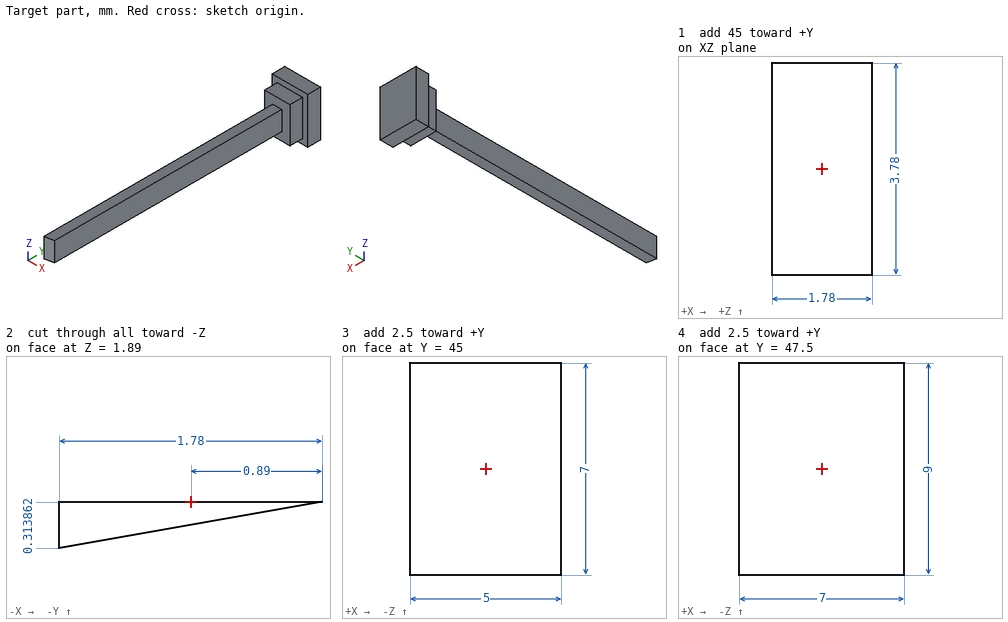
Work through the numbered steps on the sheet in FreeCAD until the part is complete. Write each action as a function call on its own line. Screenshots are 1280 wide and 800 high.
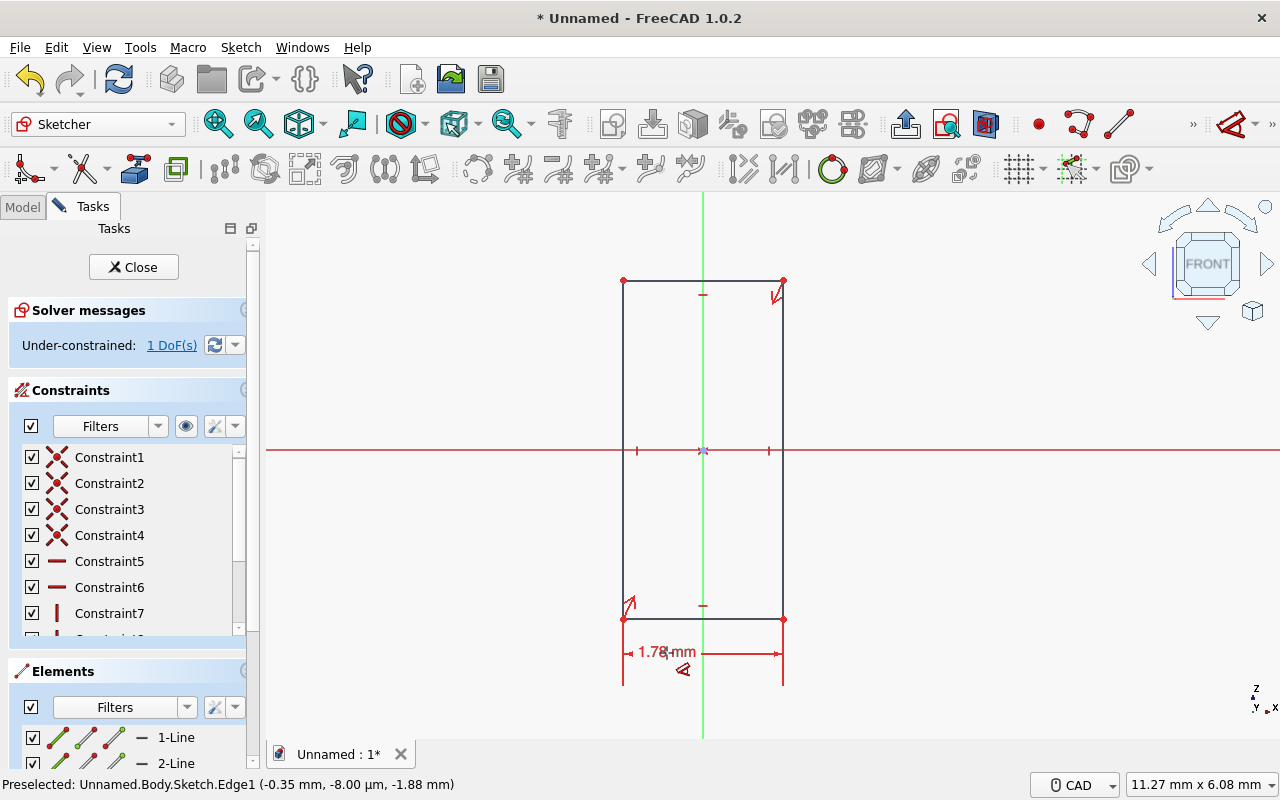
click(783, 518)
click(817, 372)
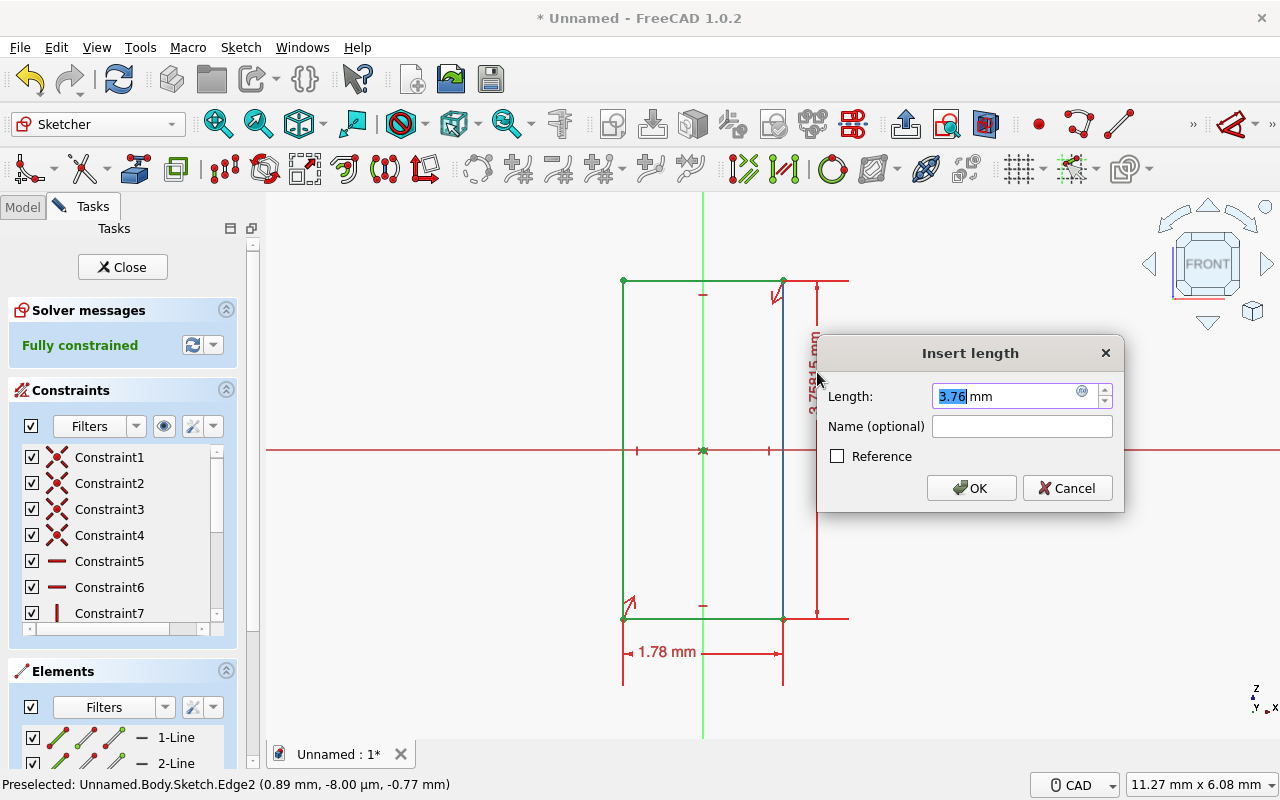
text(3.78)
key(Return)
key(Escape)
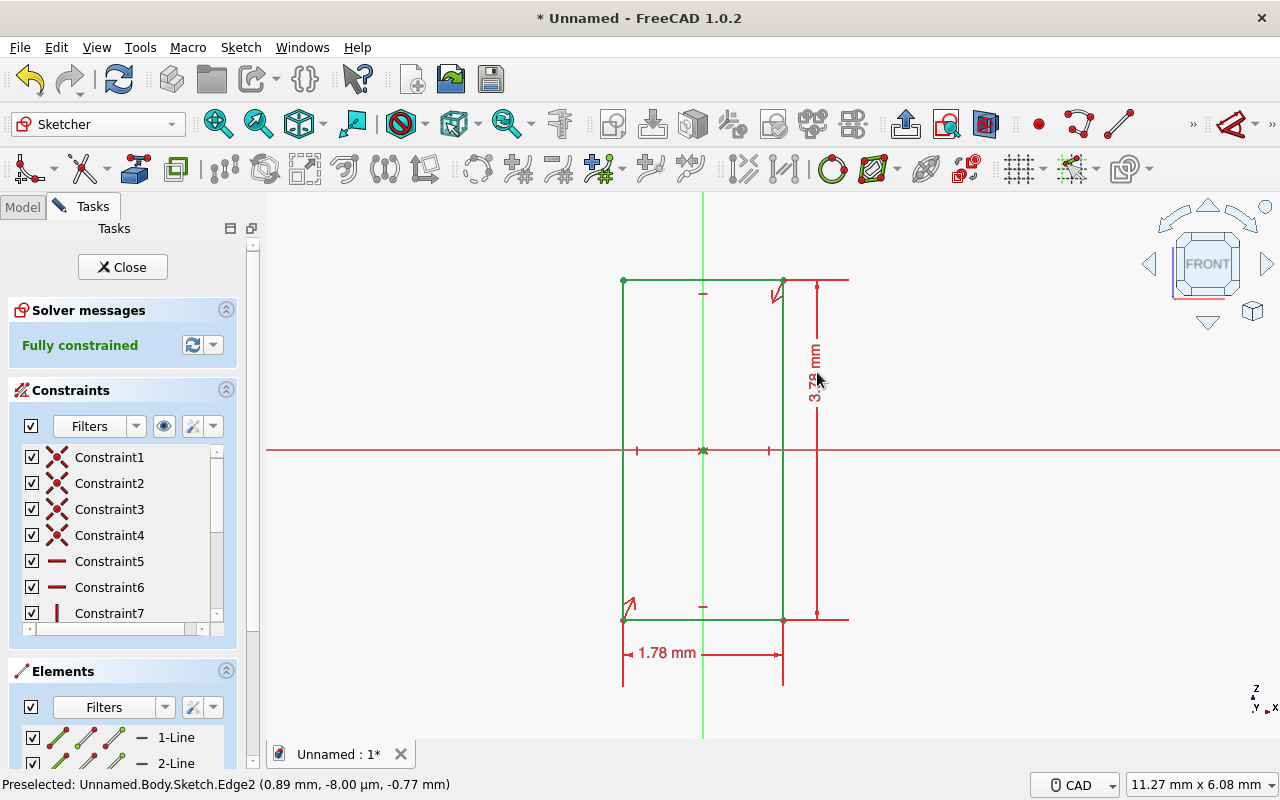
click(123, 267)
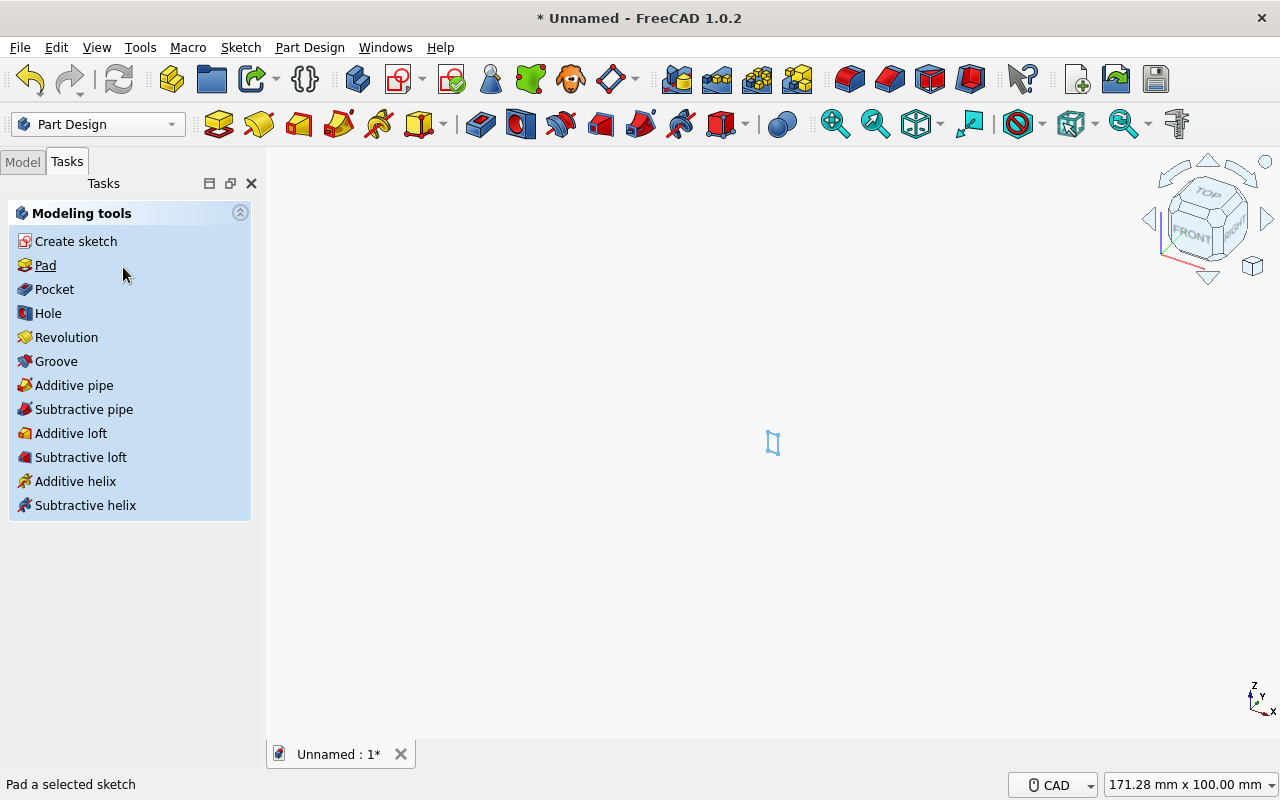
click(220, 124)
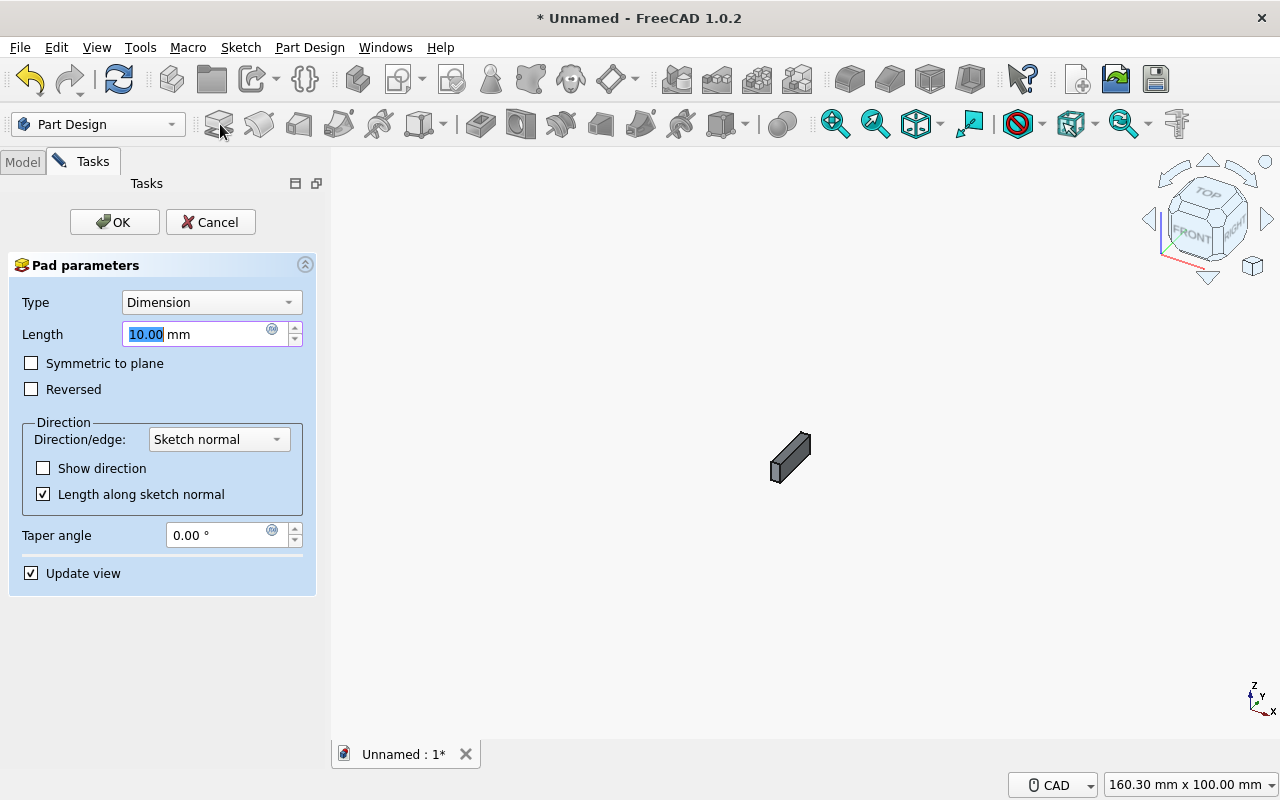
text(45)
key(Tab)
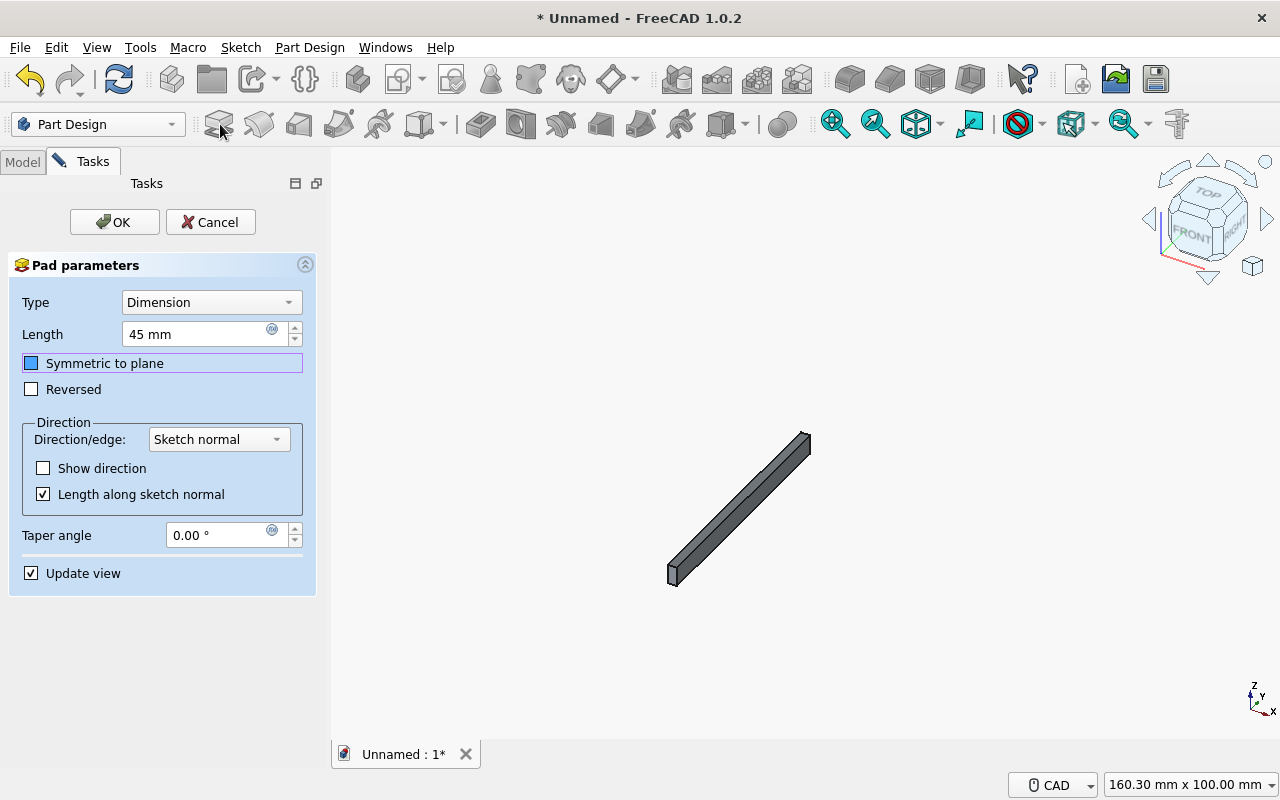
click(30, 389)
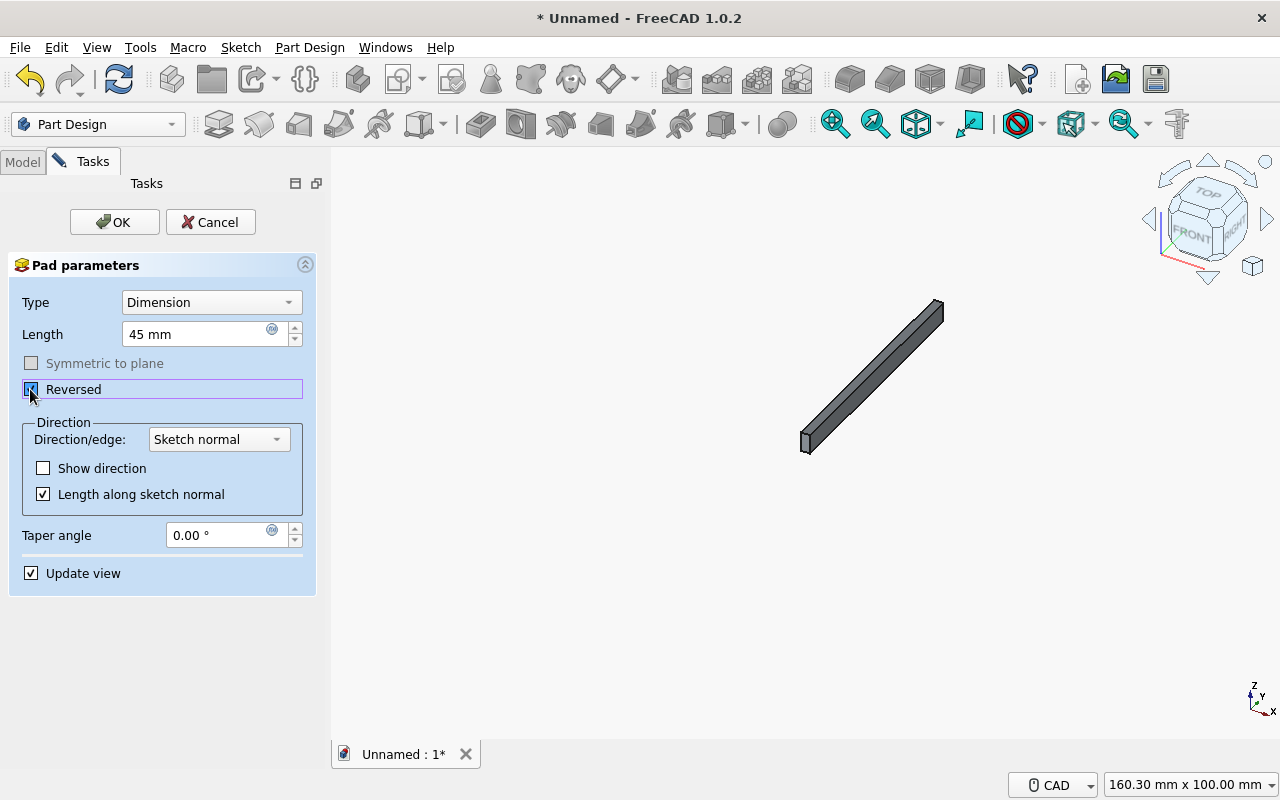
click(115, 222)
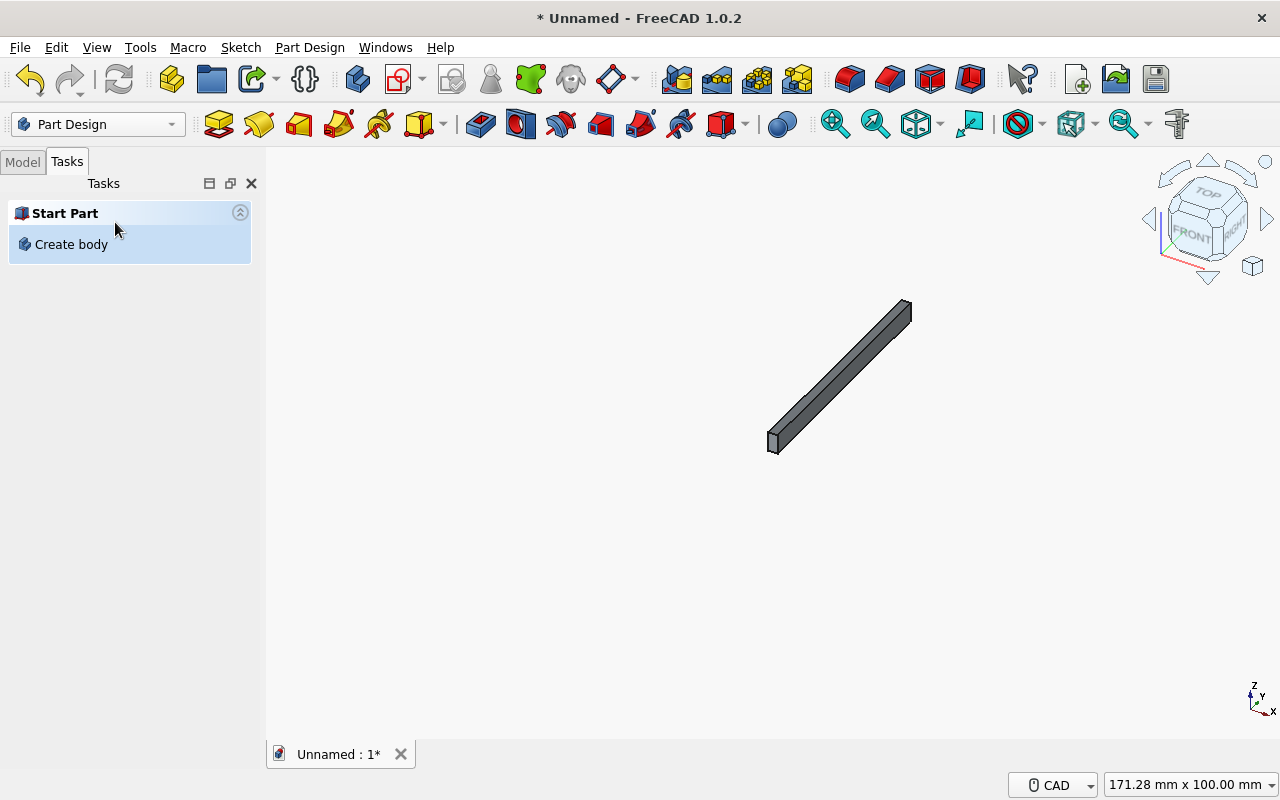
key(v)
key(f)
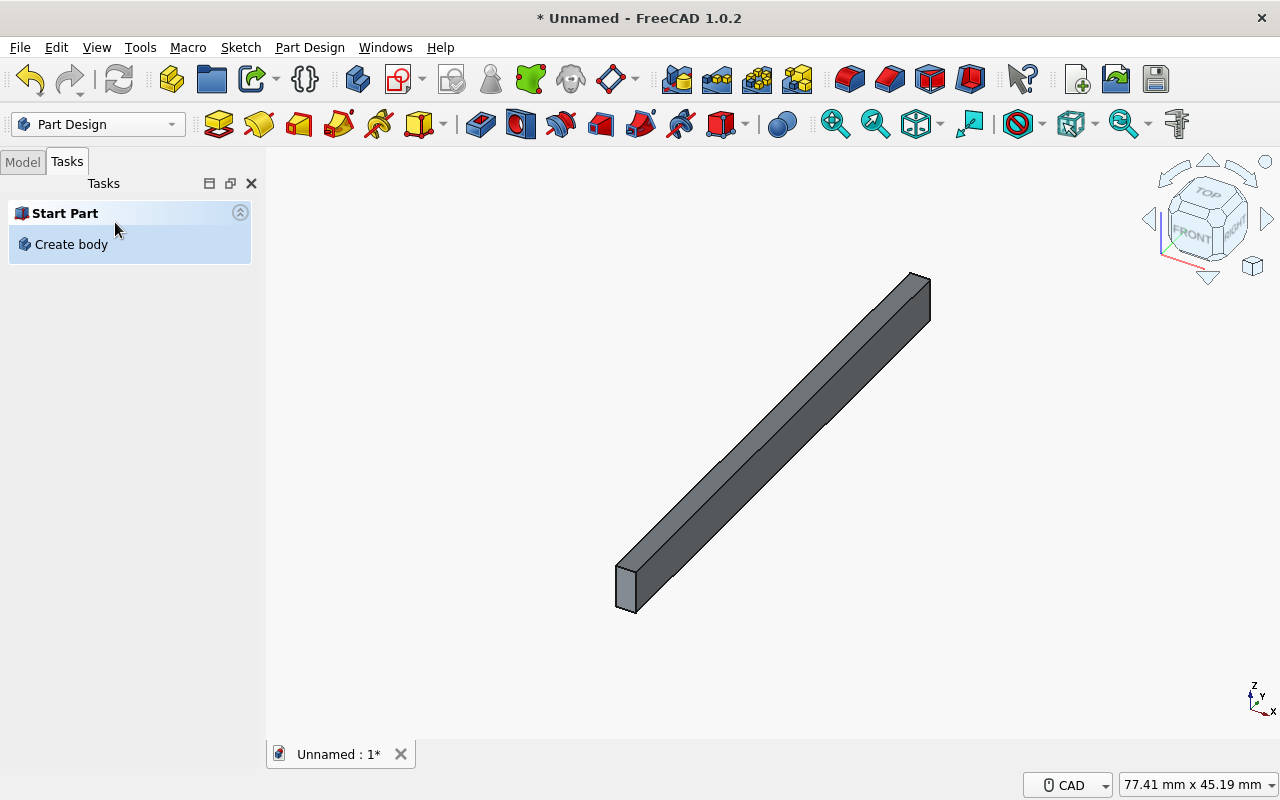
click(899, 296)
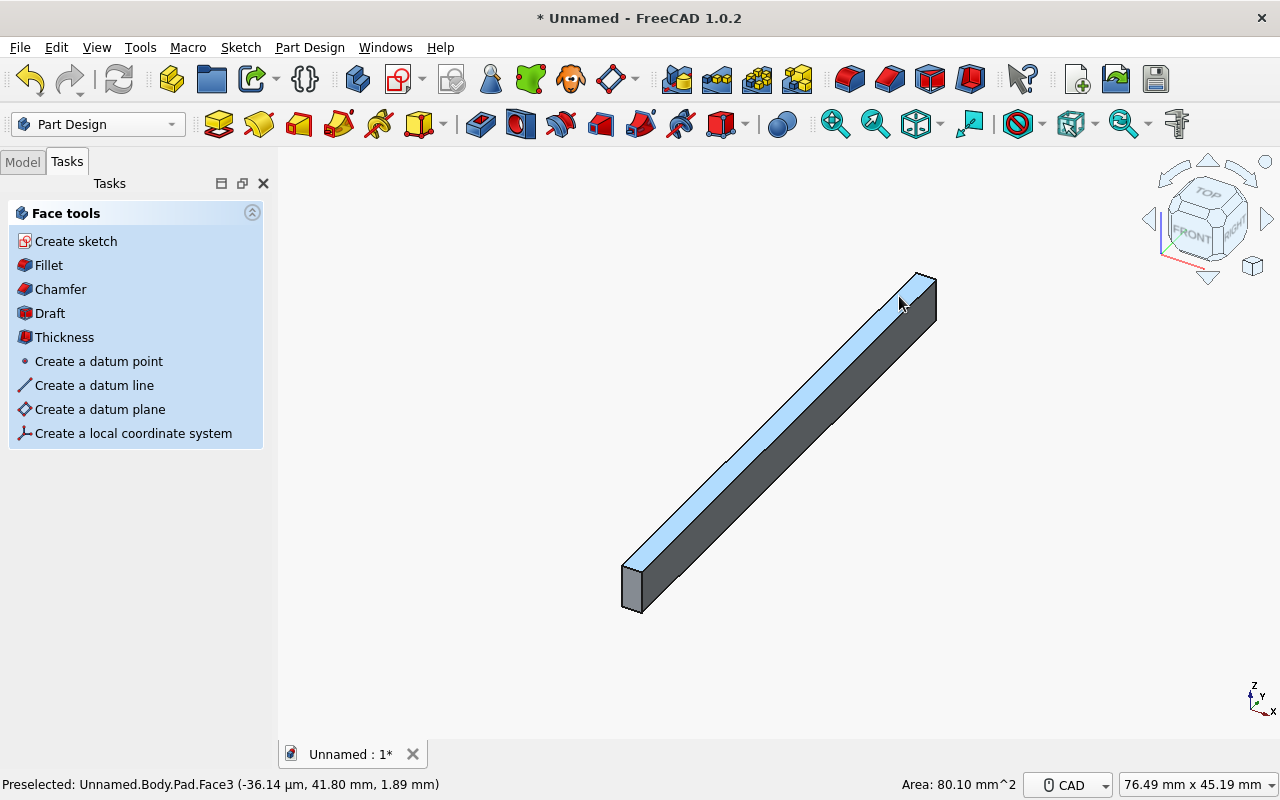
click(398, 80)